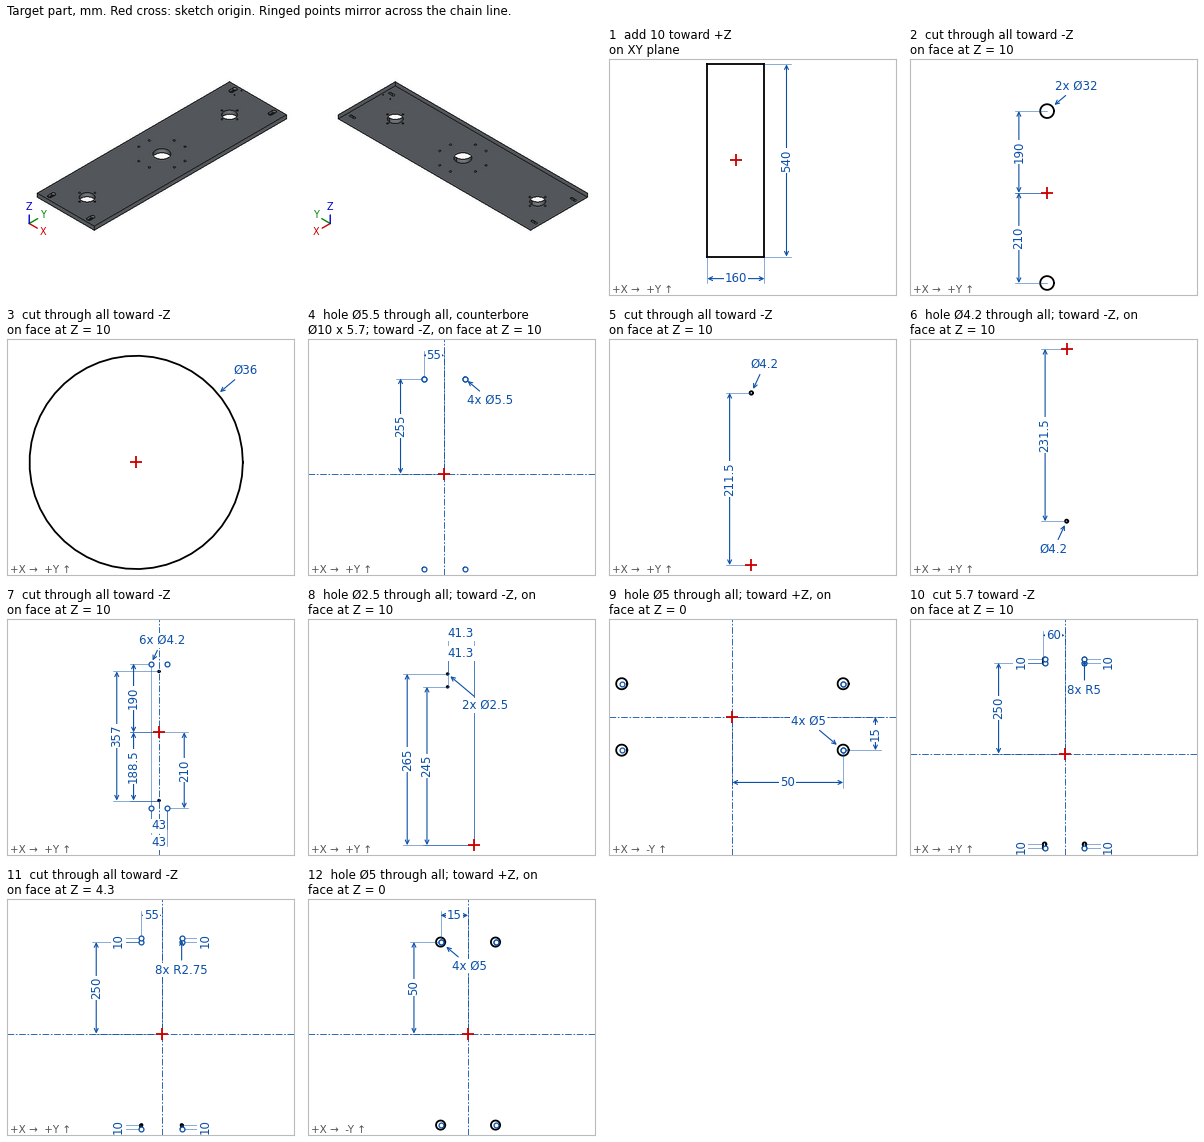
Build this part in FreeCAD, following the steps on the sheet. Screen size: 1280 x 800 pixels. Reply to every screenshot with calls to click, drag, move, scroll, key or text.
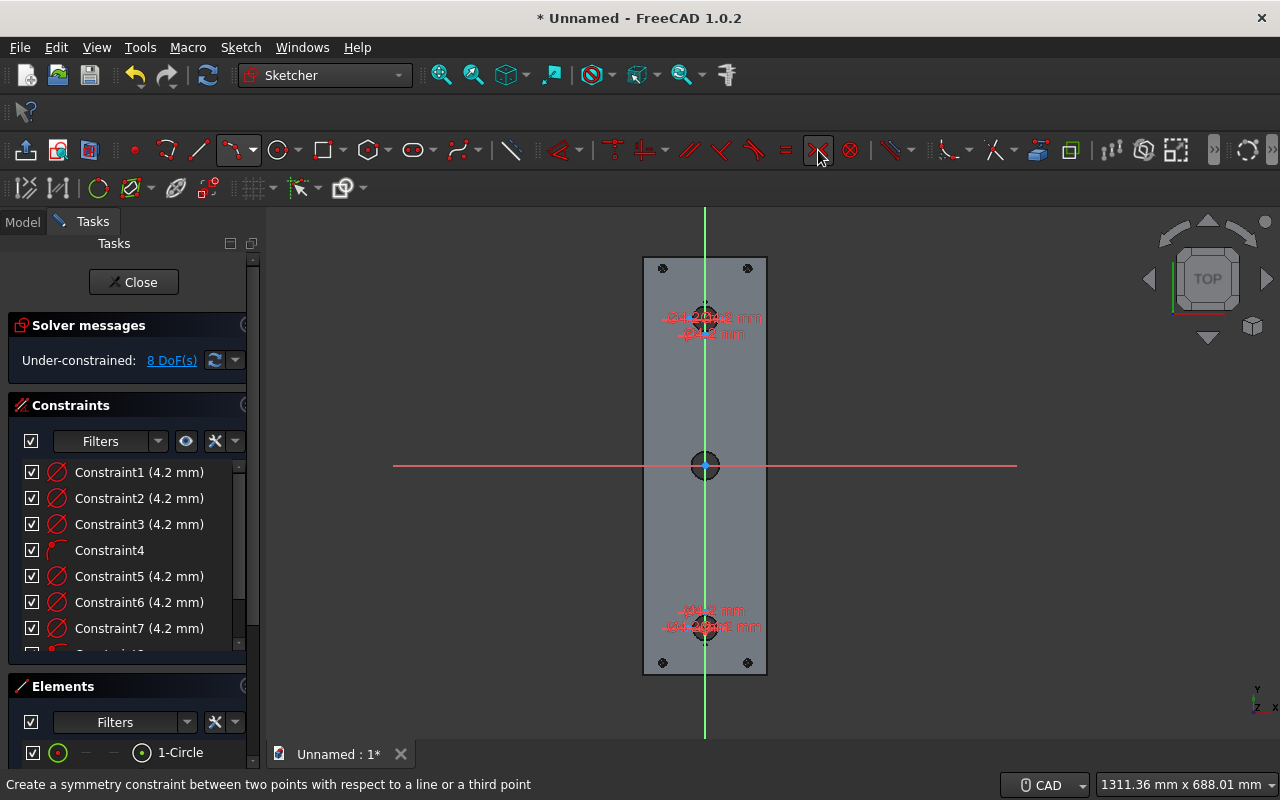
click(689, 320)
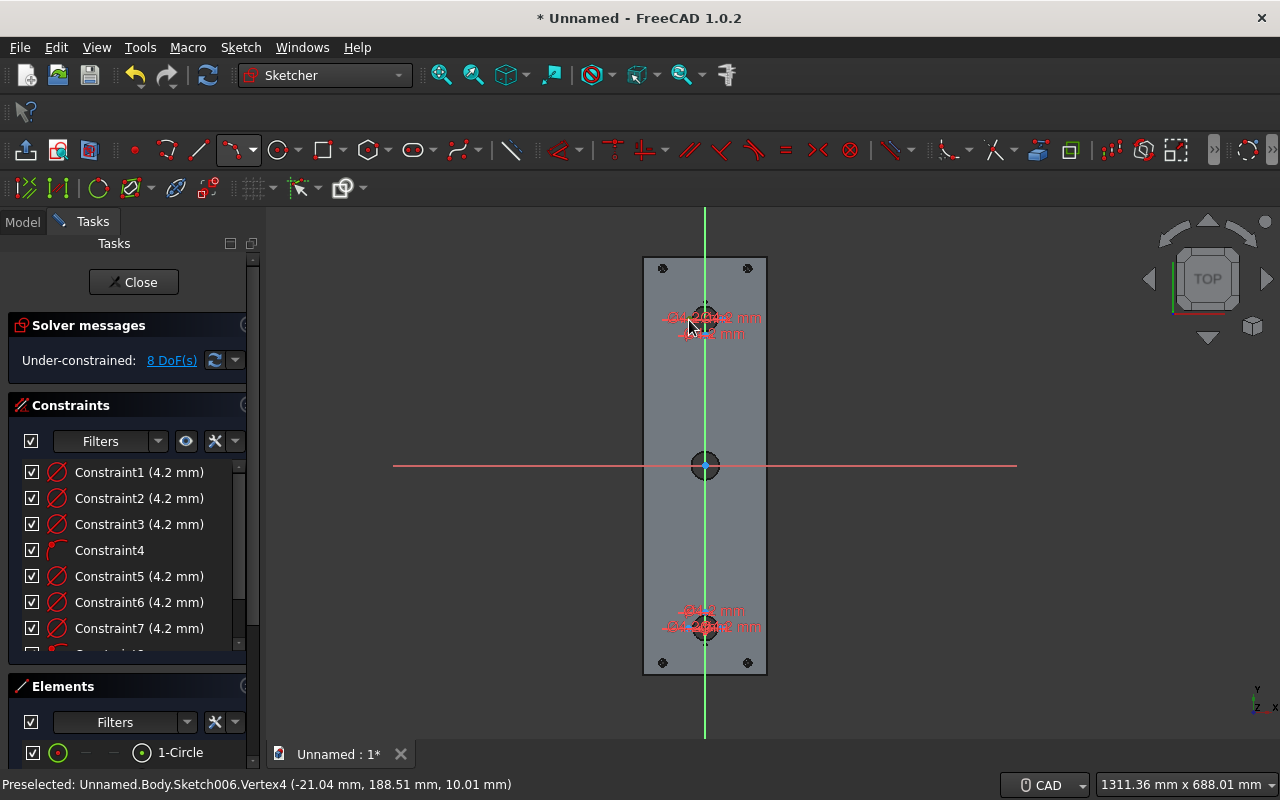
click(722, 320)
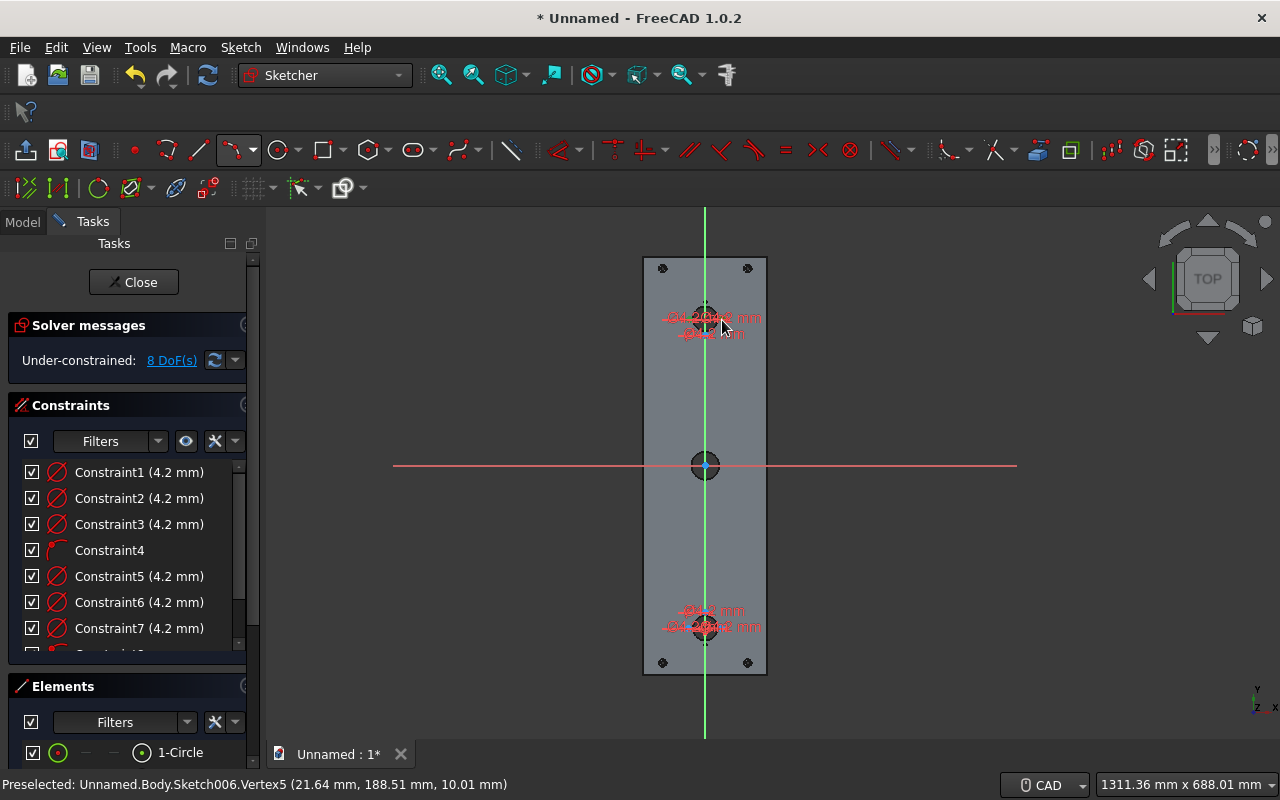
click(705, 677)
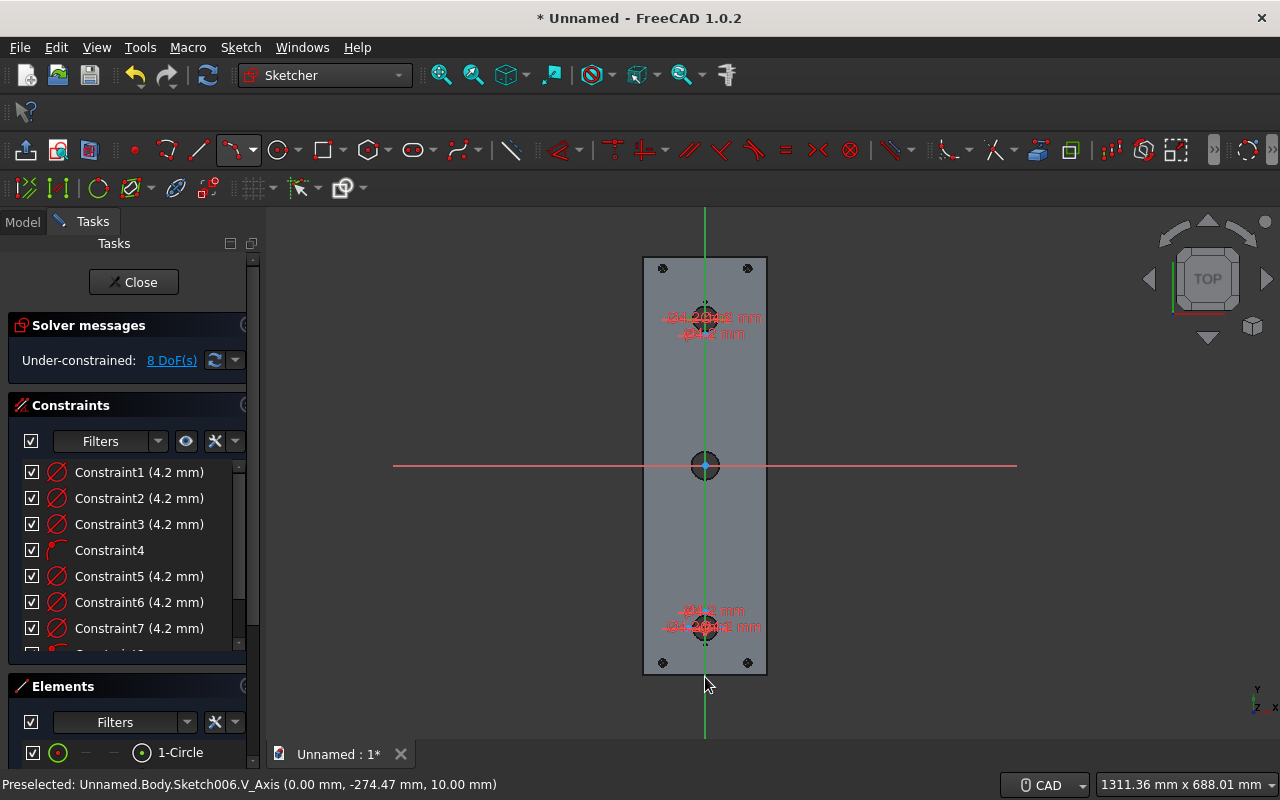
click(818, 150)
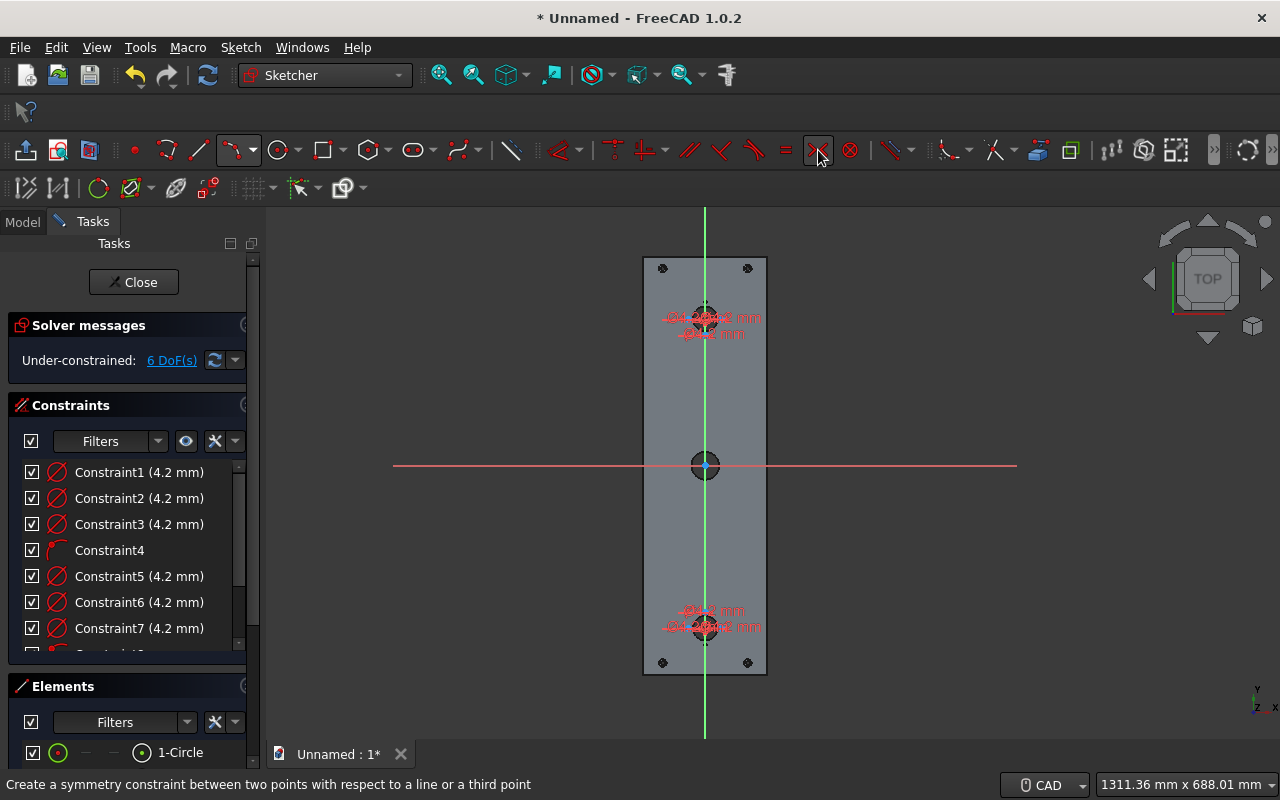
click(558, 150)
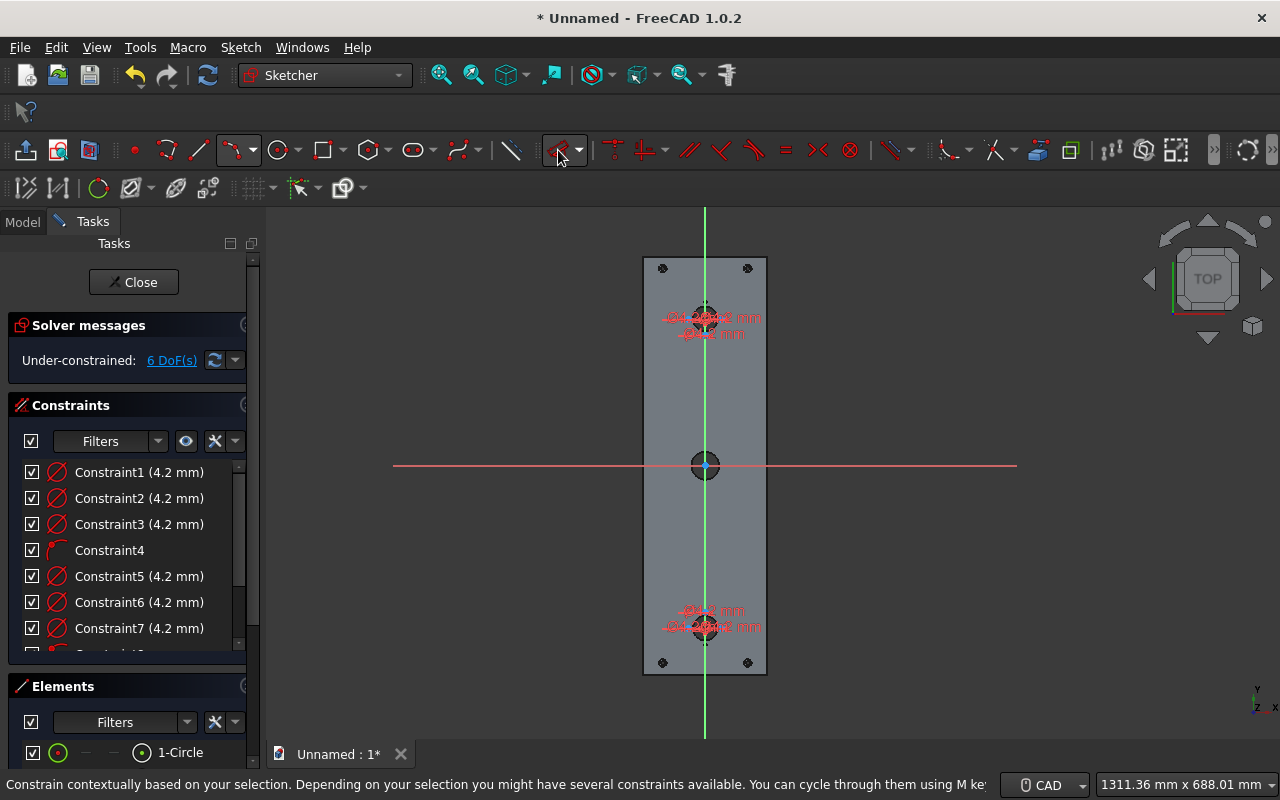
click(722, 629)
click(756, 547)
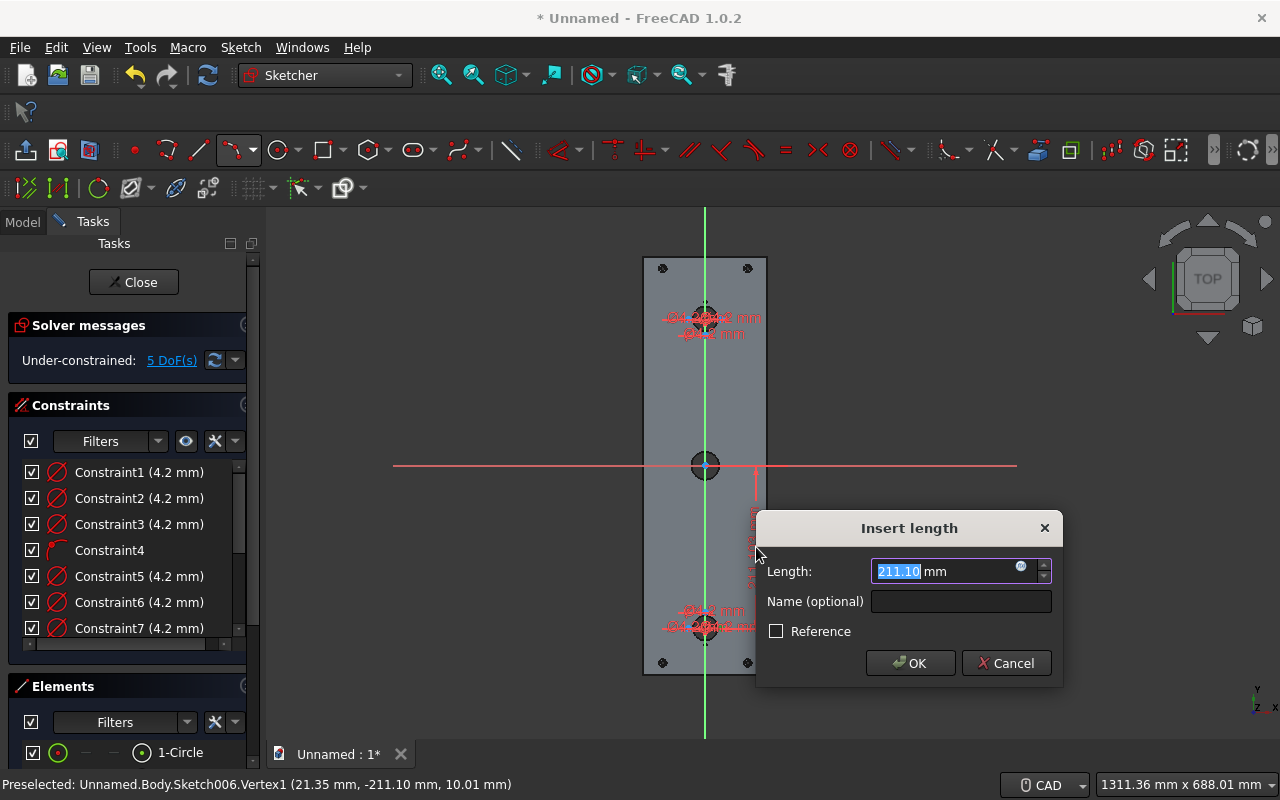
text(210)
key(Return)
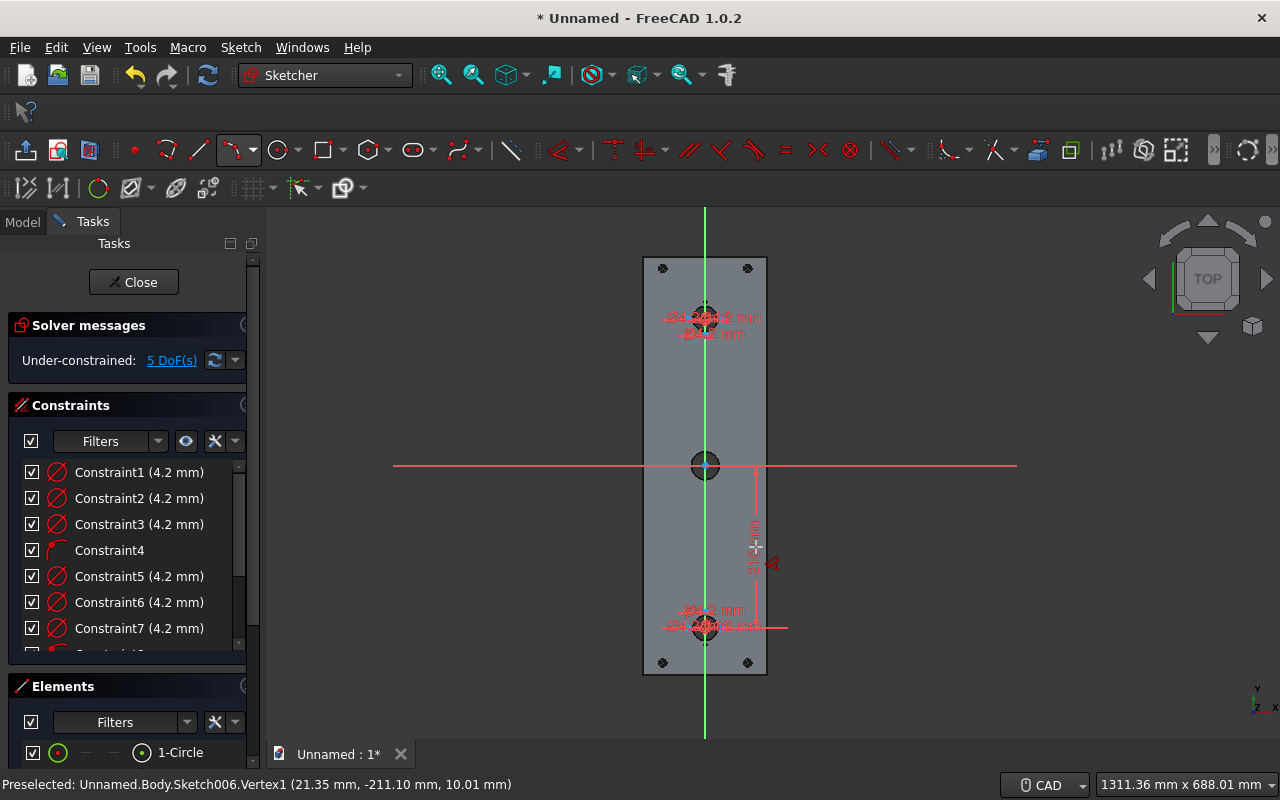
click(689, 320)
click(655, 393)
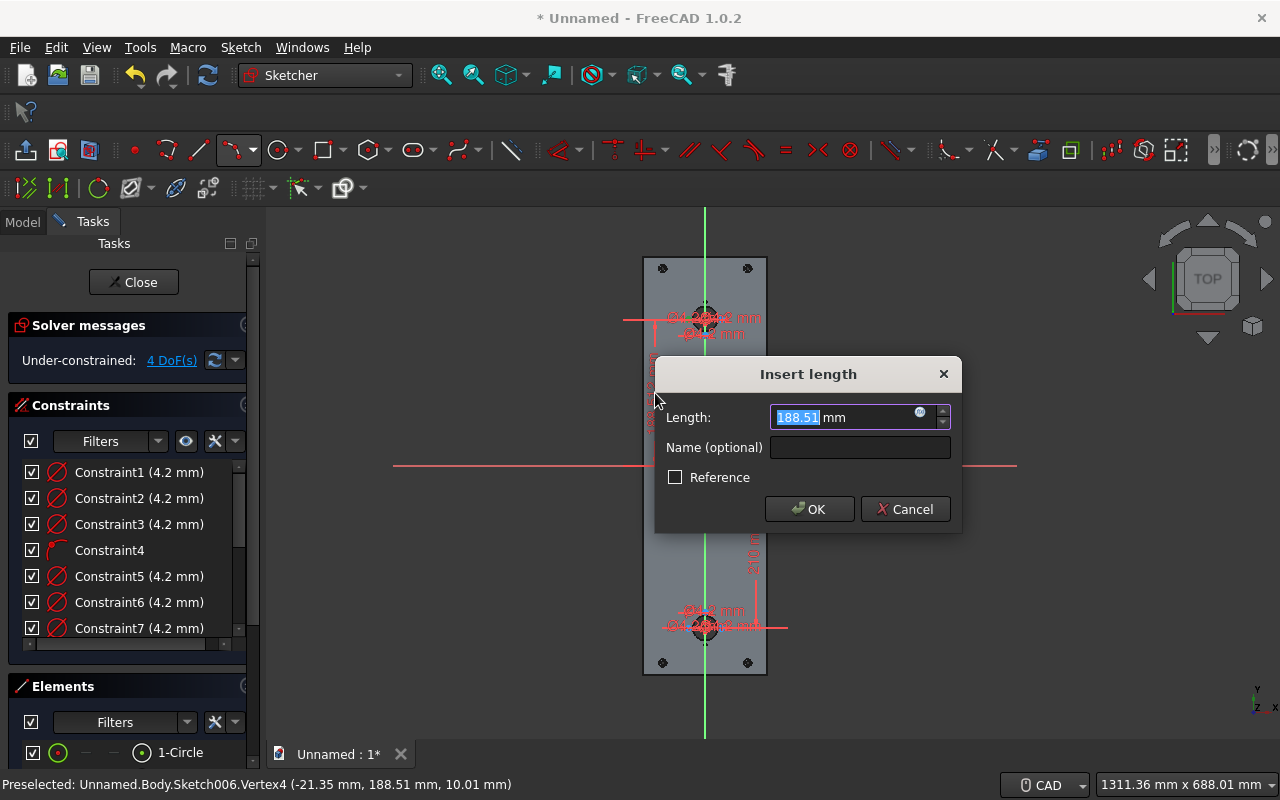
text(190)
key(Return)